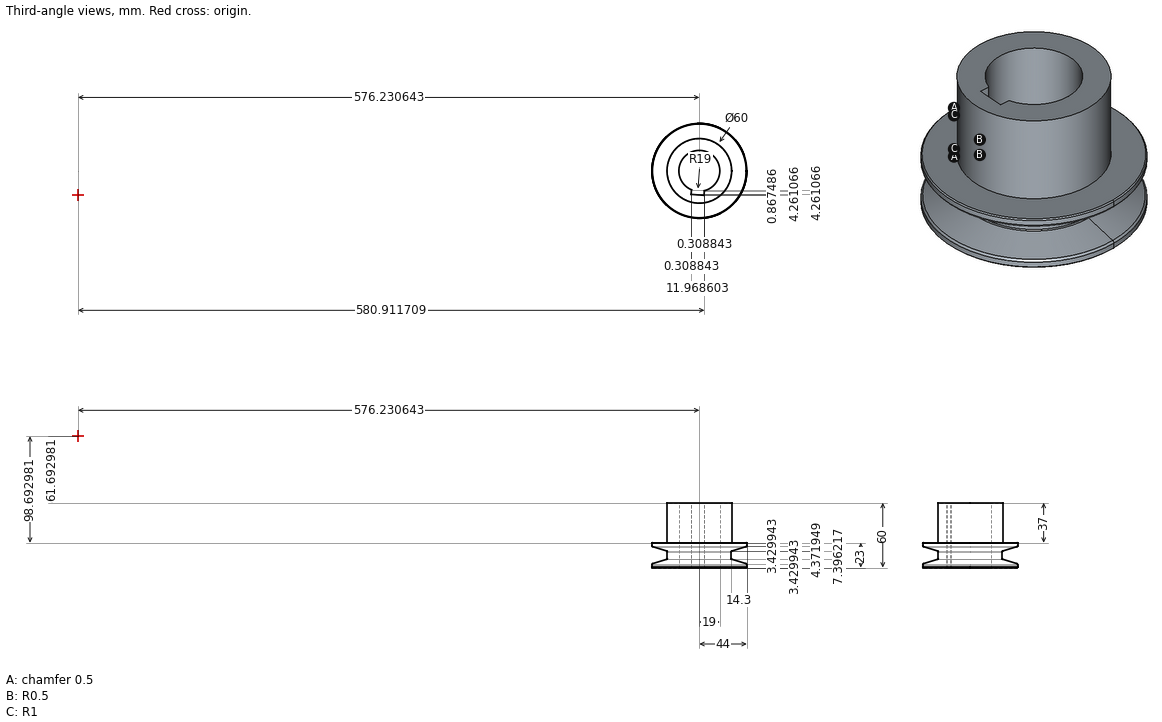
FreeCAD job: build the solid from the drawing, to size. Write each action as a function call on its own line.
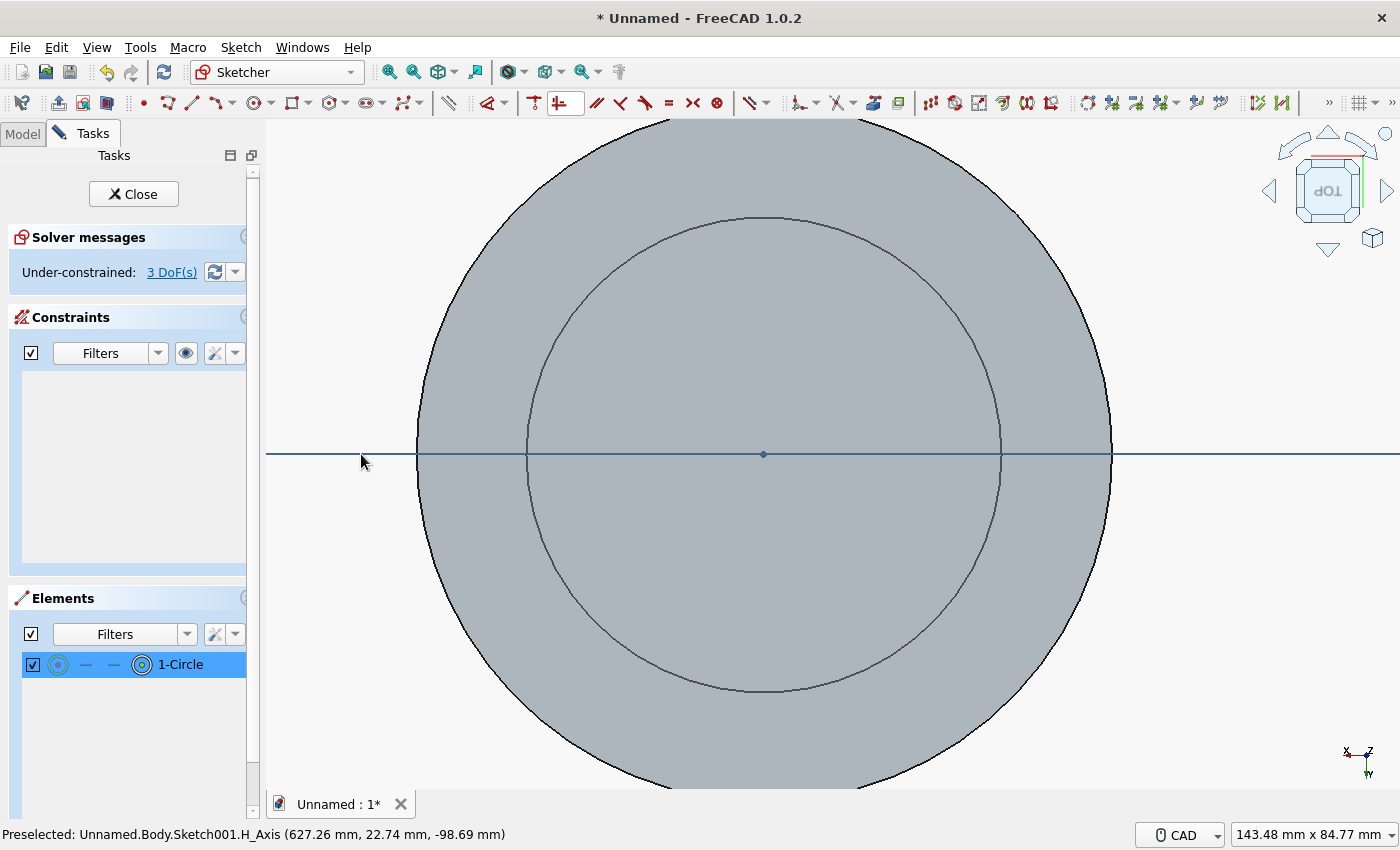
click(534, 104)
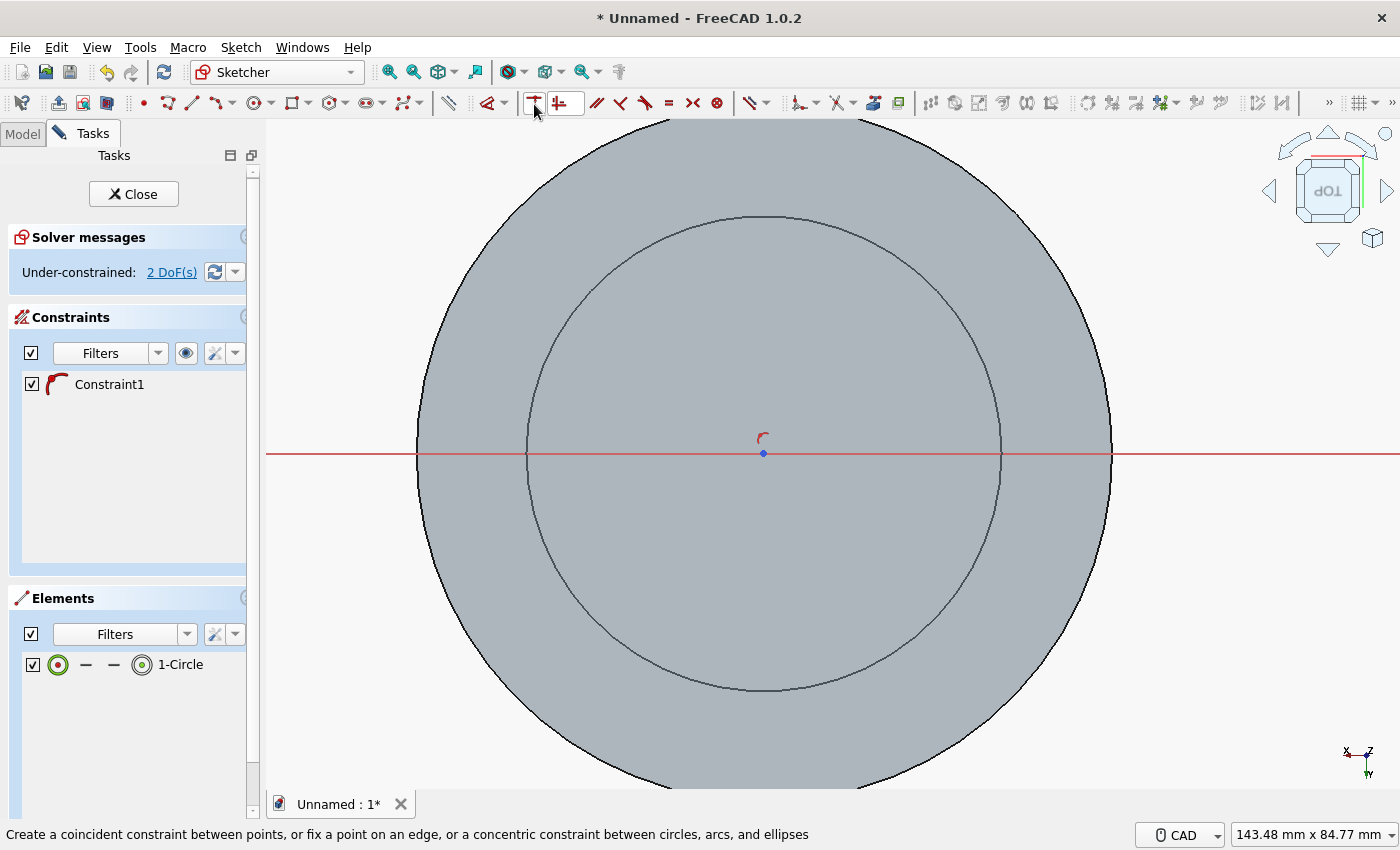
click(488, 104)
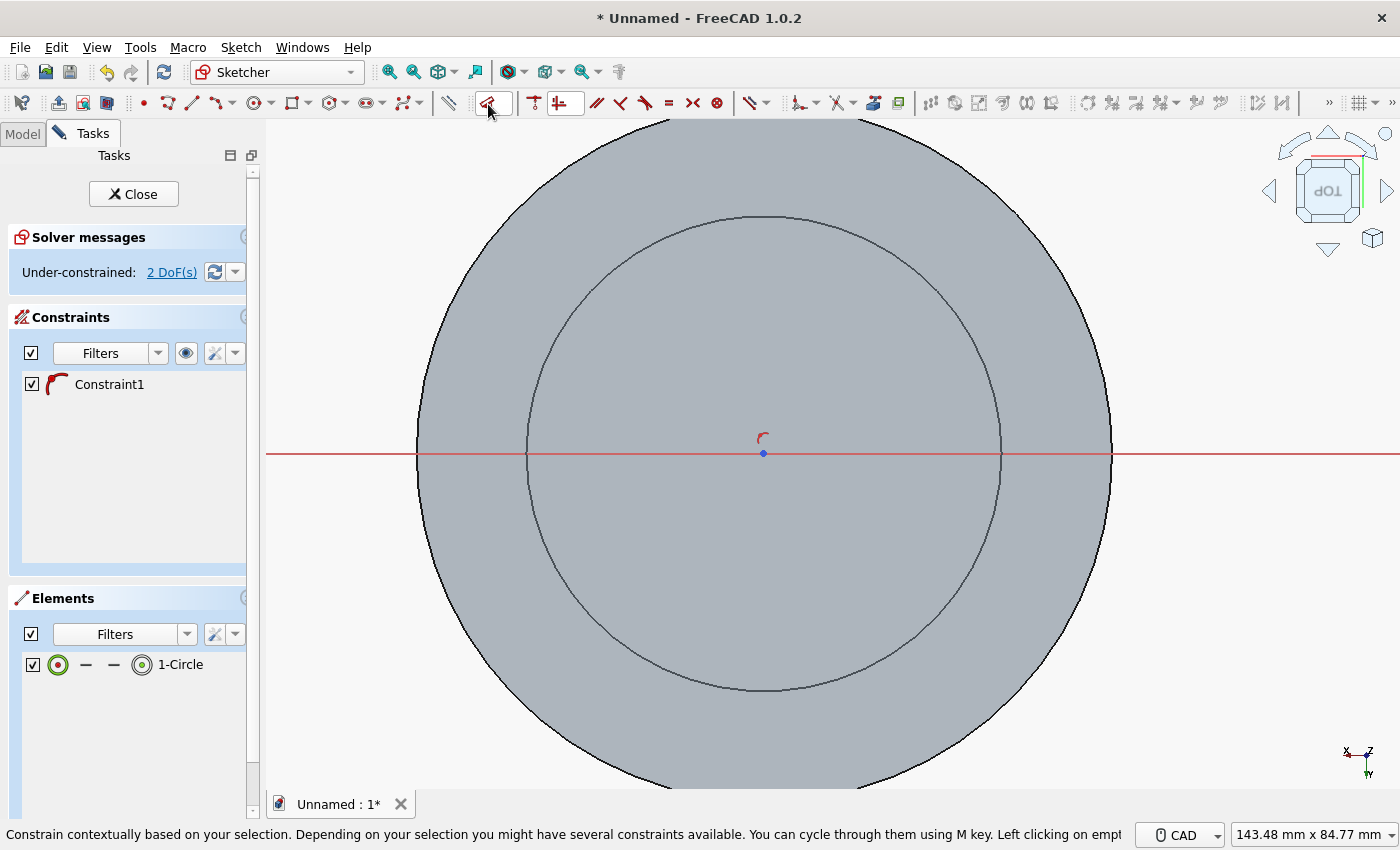
click(931, 285)
click(954, 262)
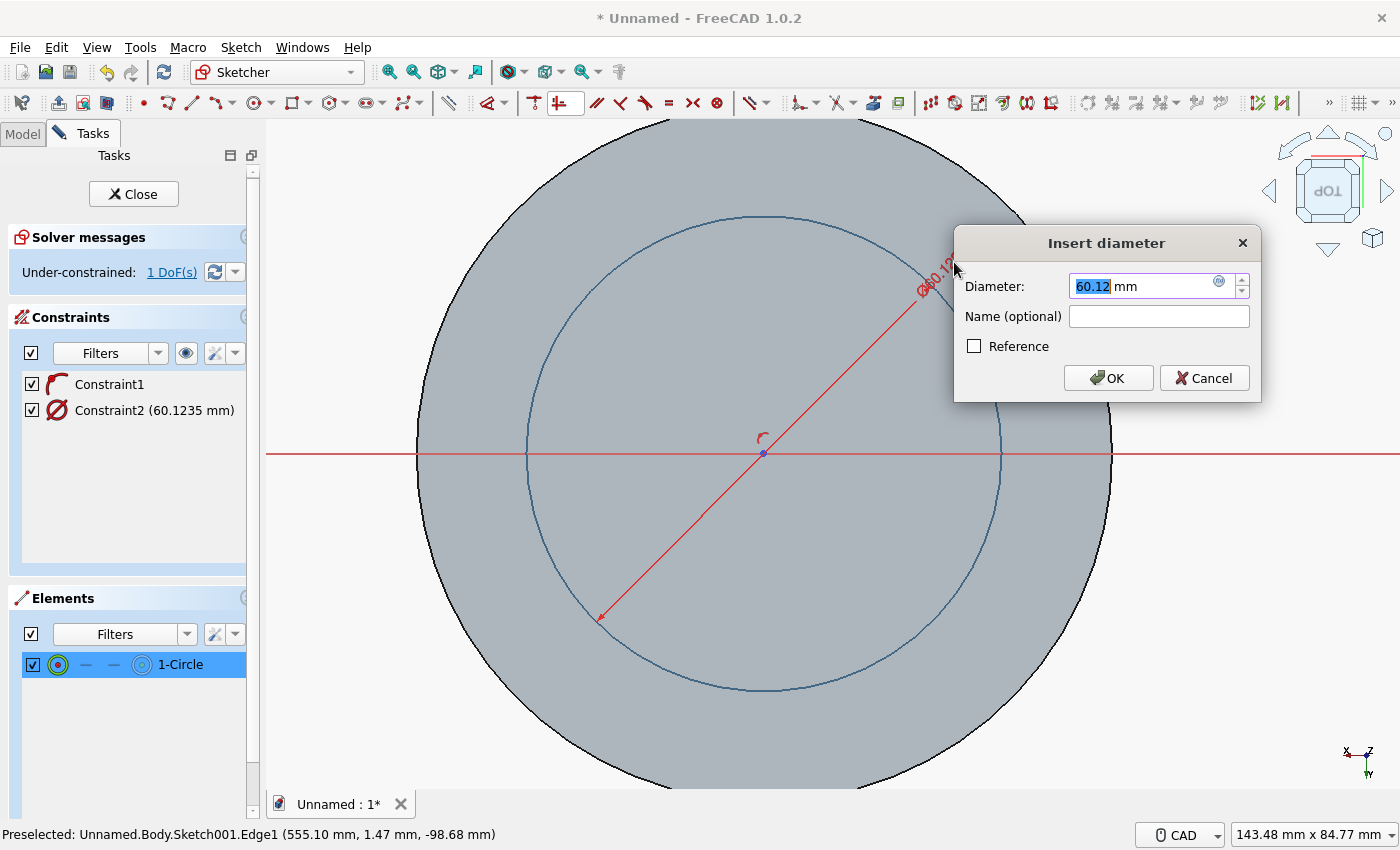
text(60)
key(Return)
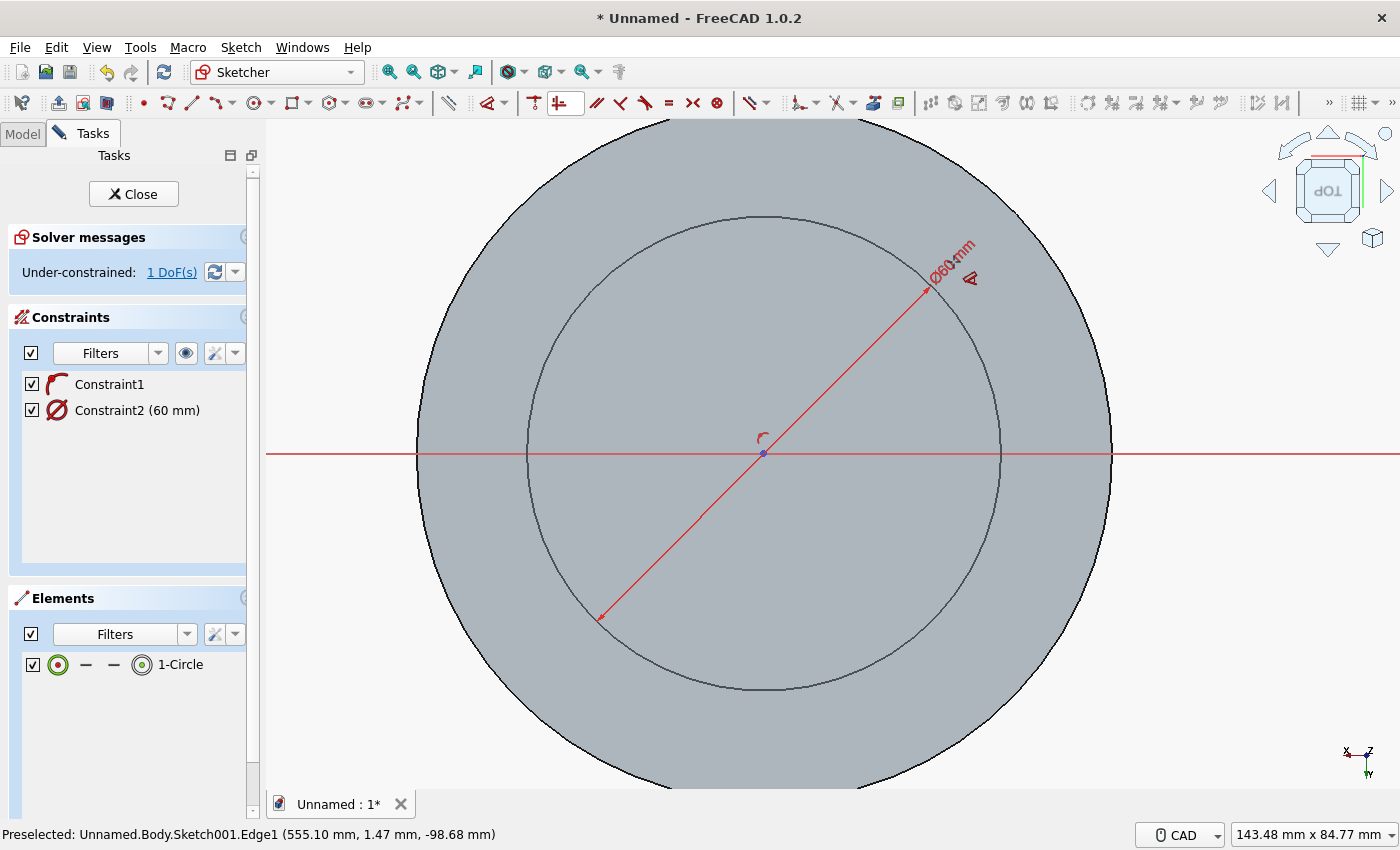
click(764, 454)
click(891, 488)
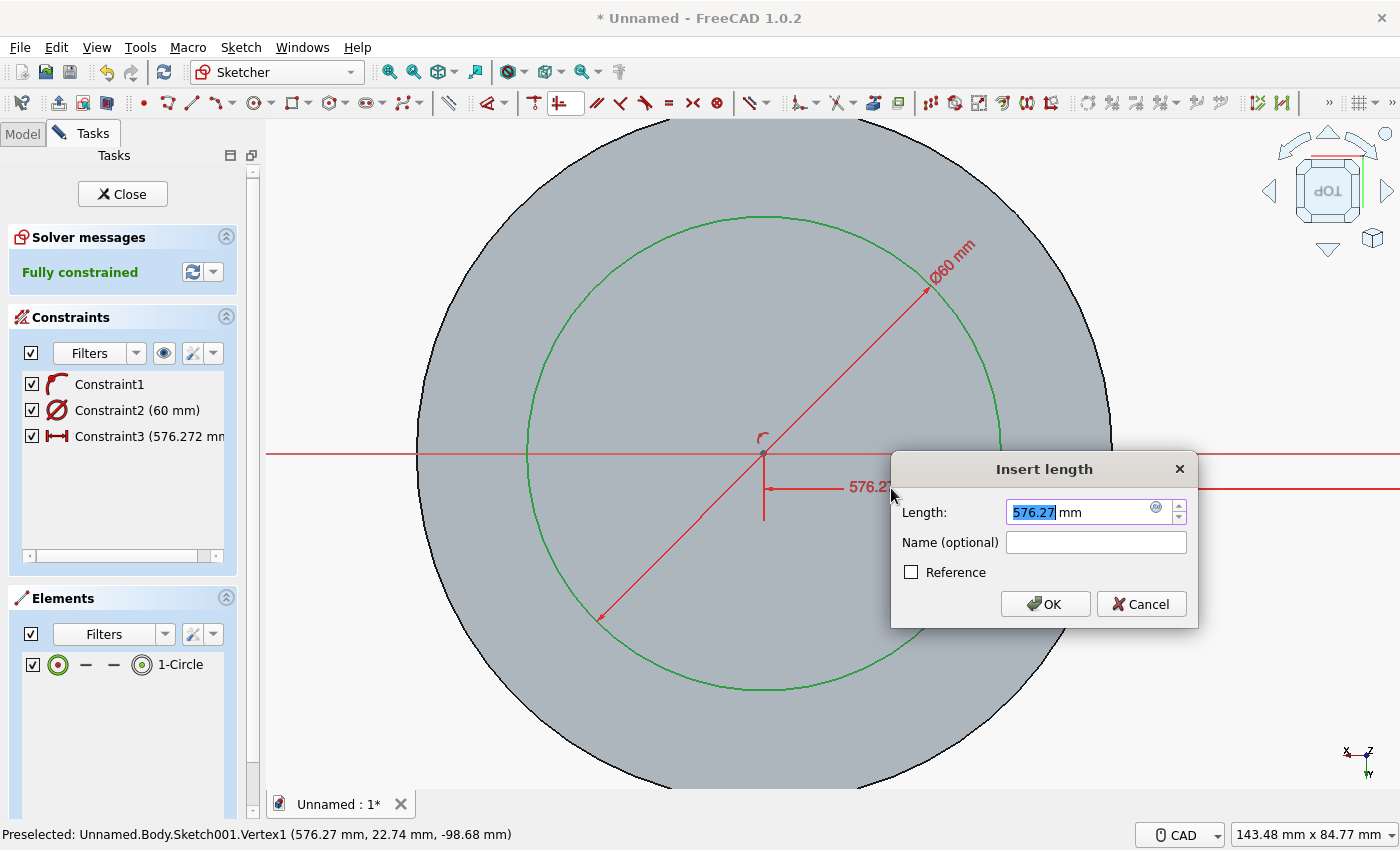
text(576.230643)
key(Return)
key(Escape)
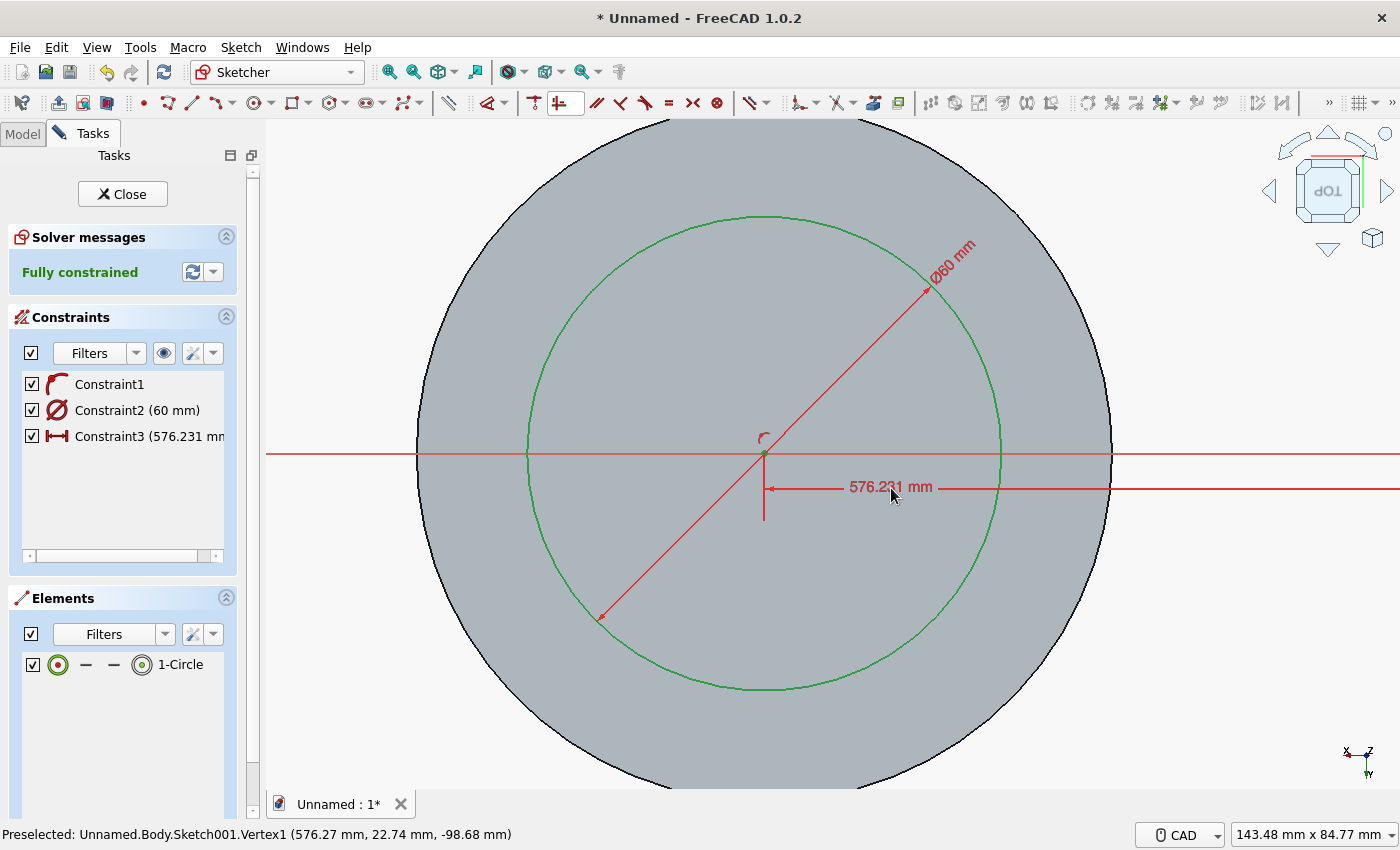
click(123, 194)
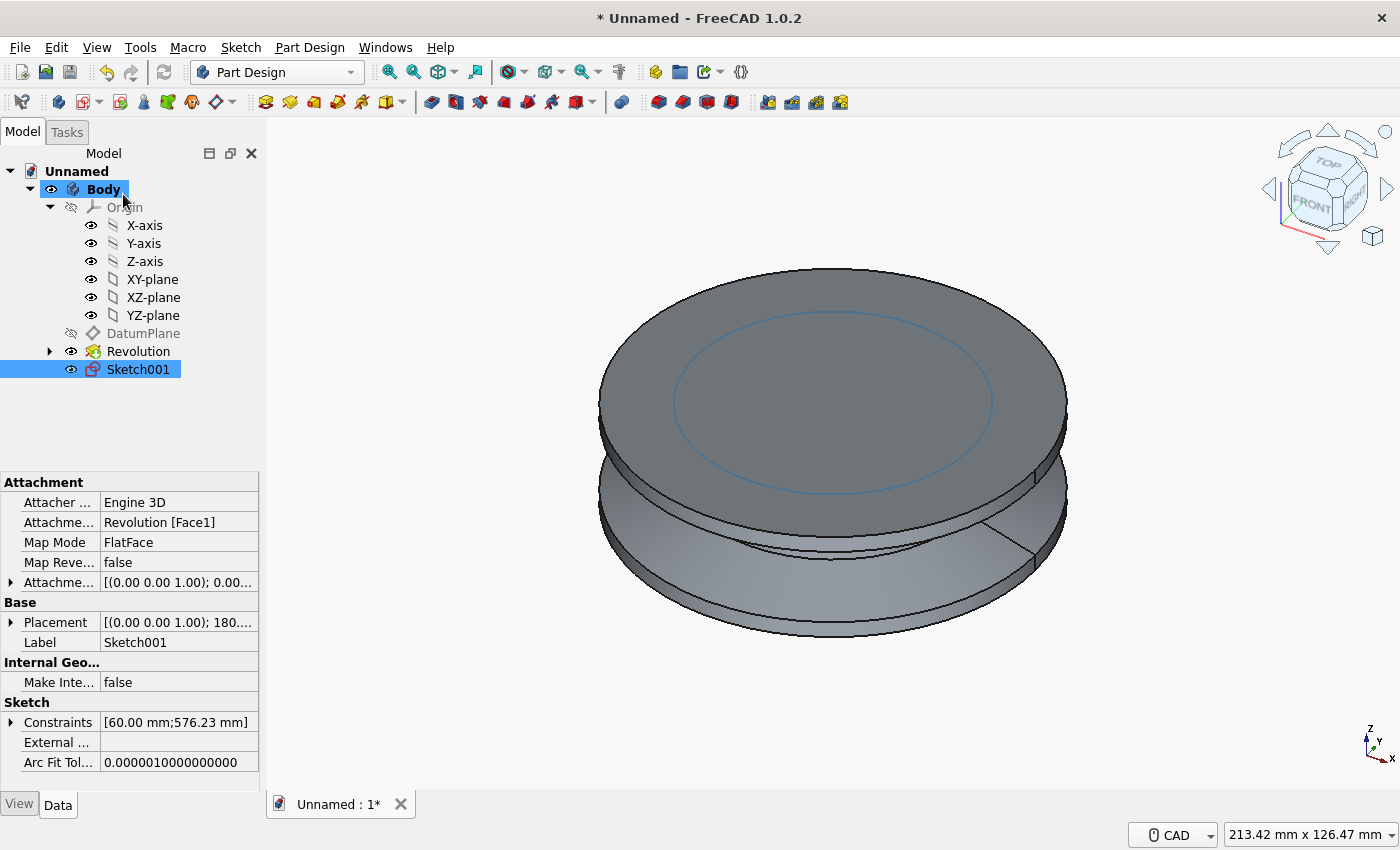
click(266, 102)